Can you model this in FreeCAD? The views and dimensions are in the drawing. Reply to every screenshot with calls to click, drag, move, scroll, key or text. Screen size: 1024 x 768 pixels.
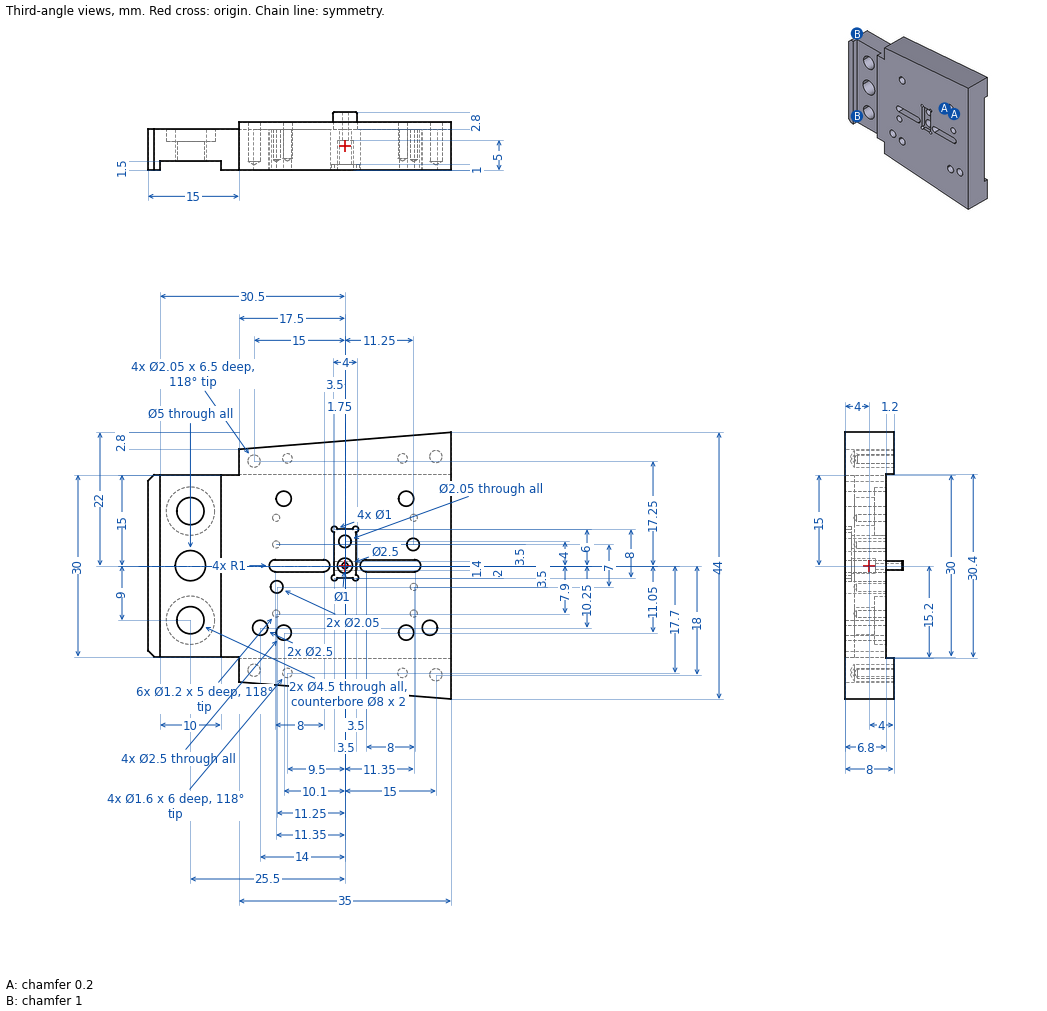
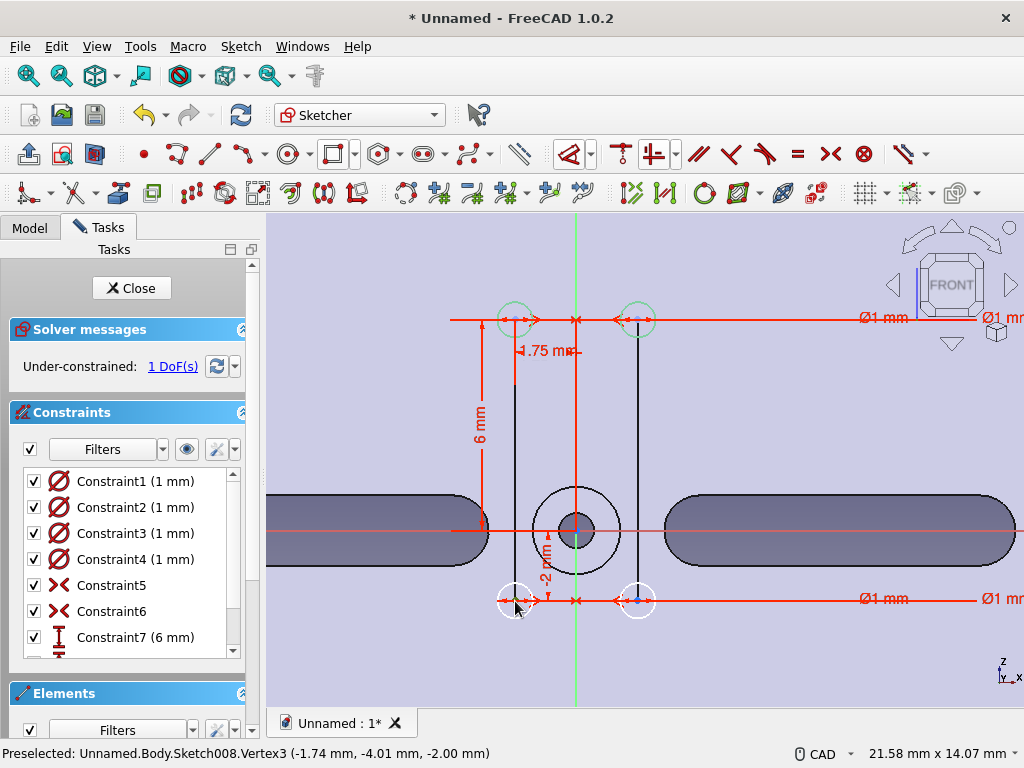
key(l)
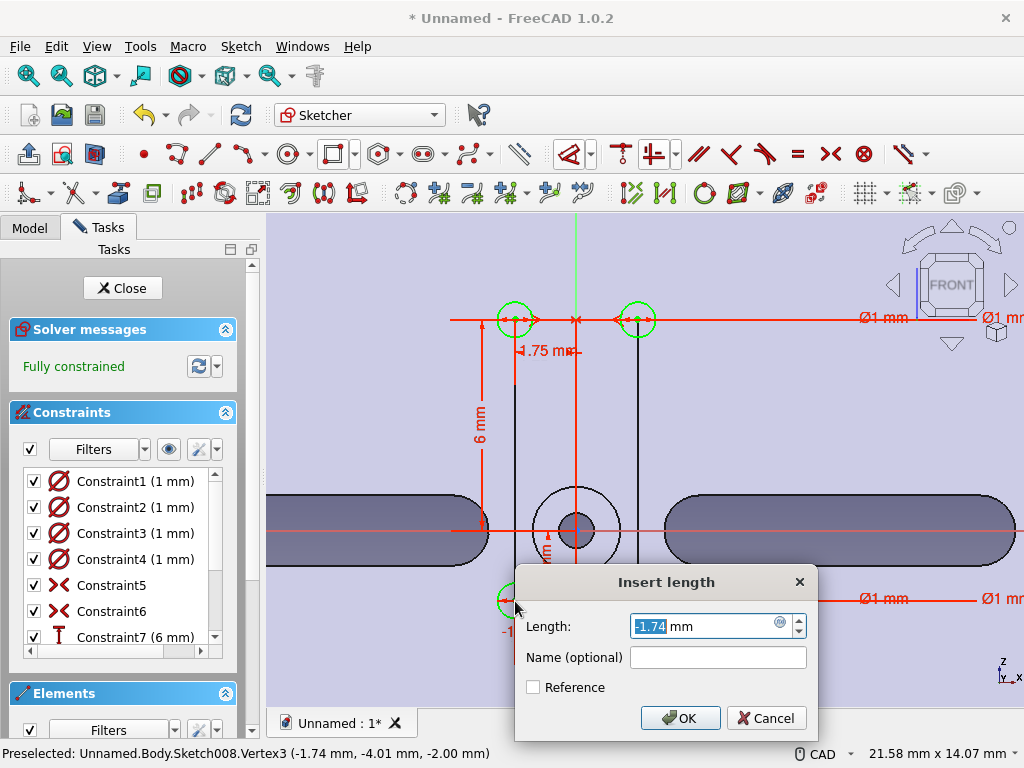
text(-1.75)
key(Return)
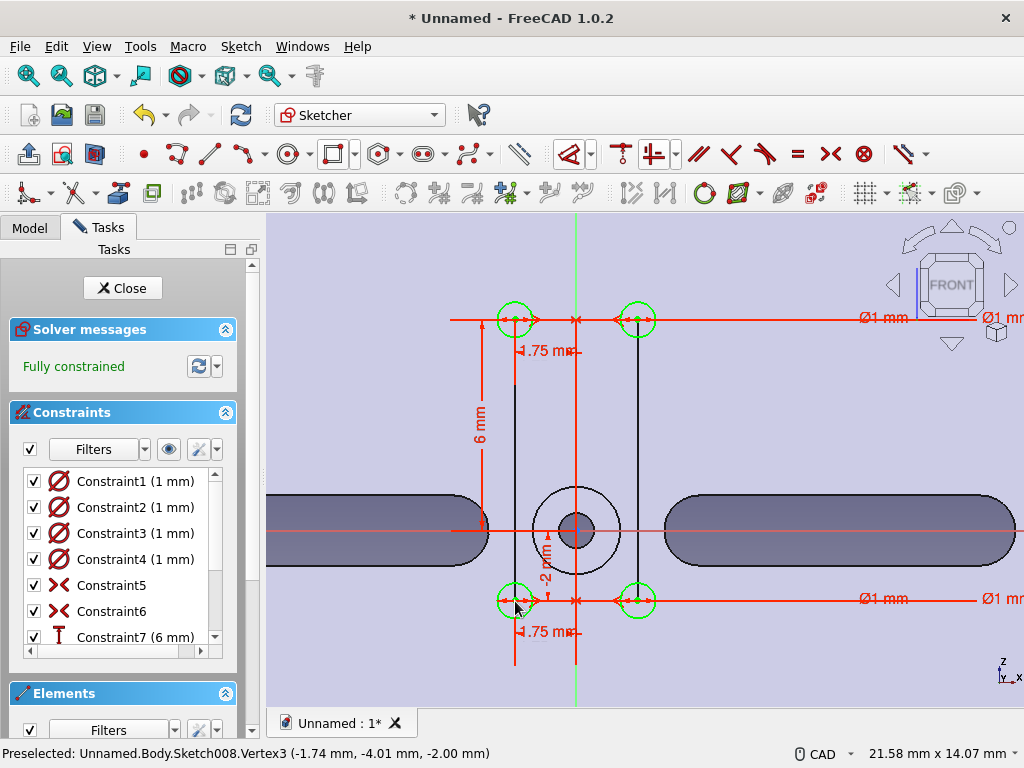
click(123, 288)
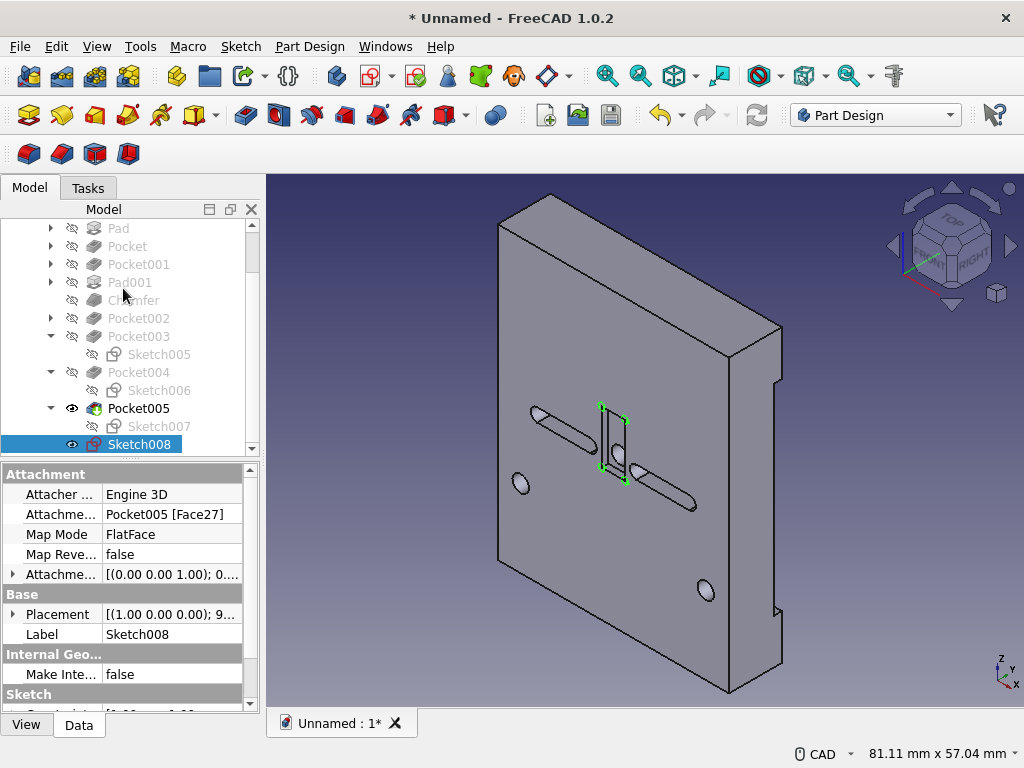
click(246, 116)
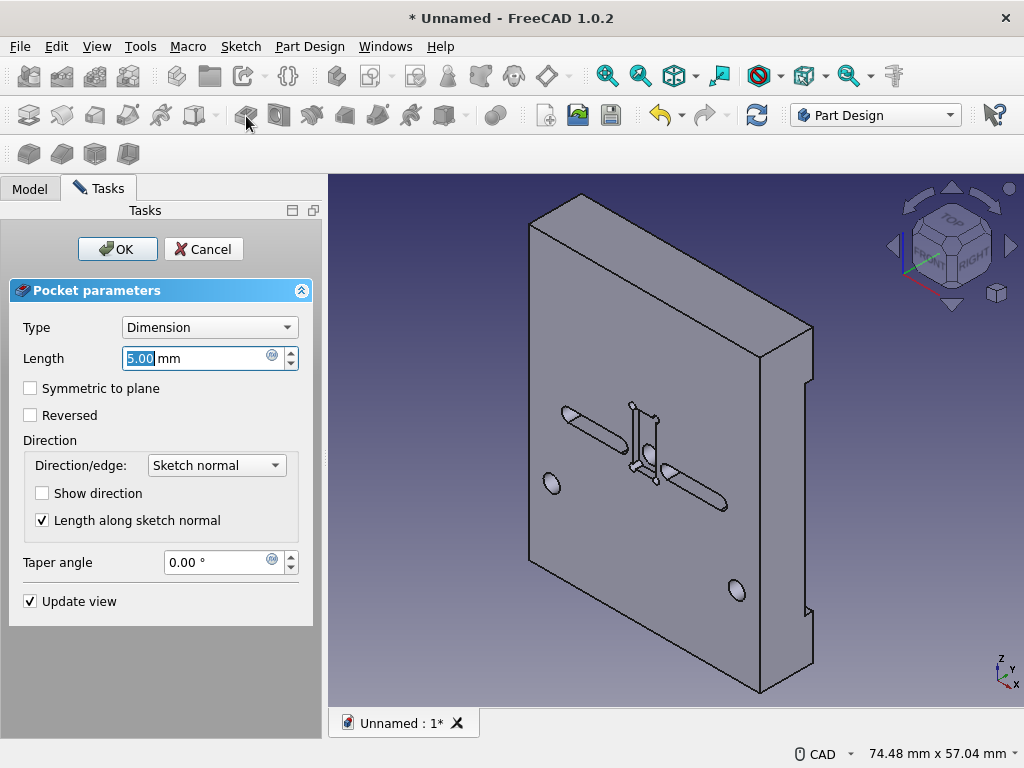
text(1)
key(Tab)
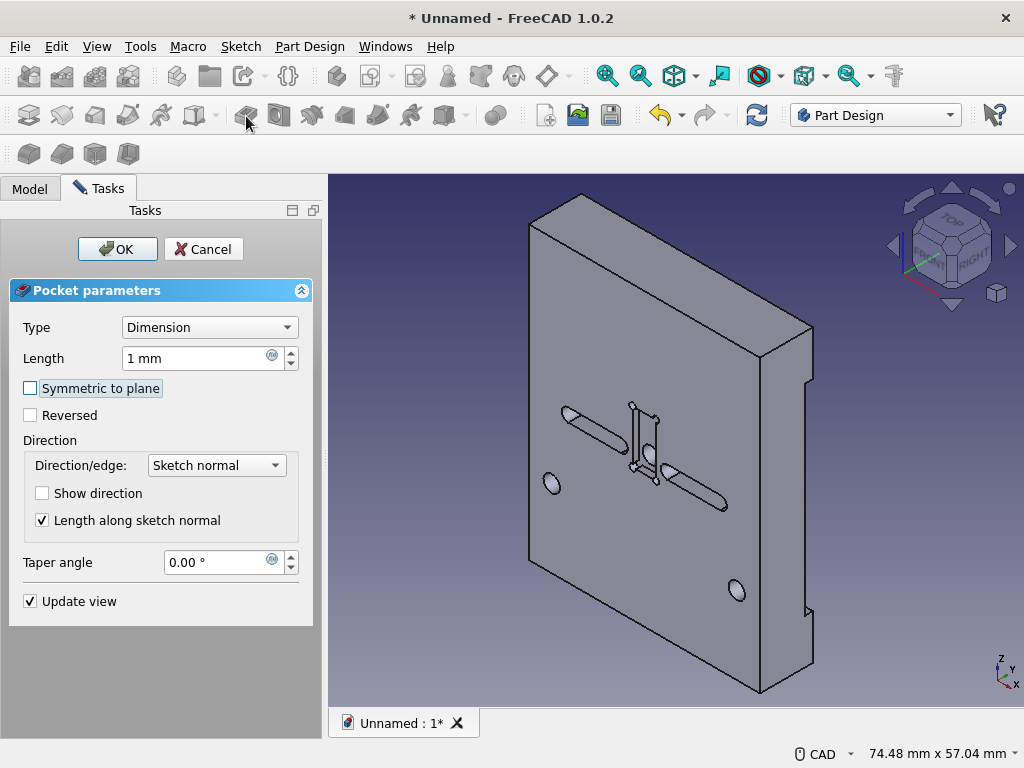
click(118, 249)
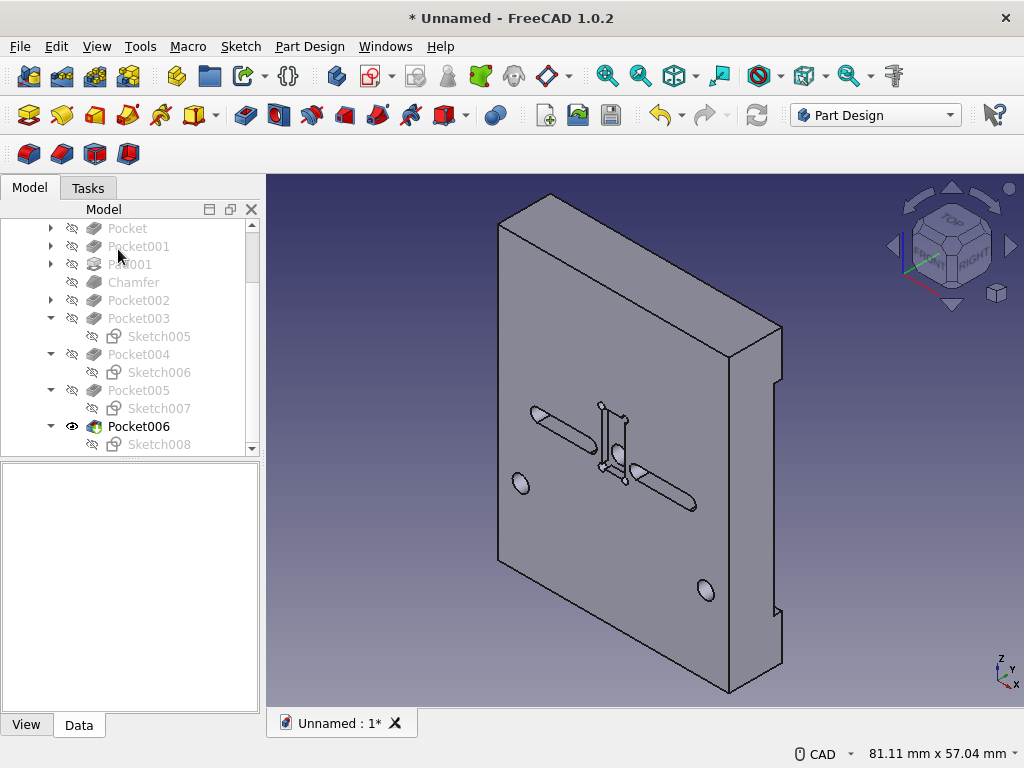
click(616, 426)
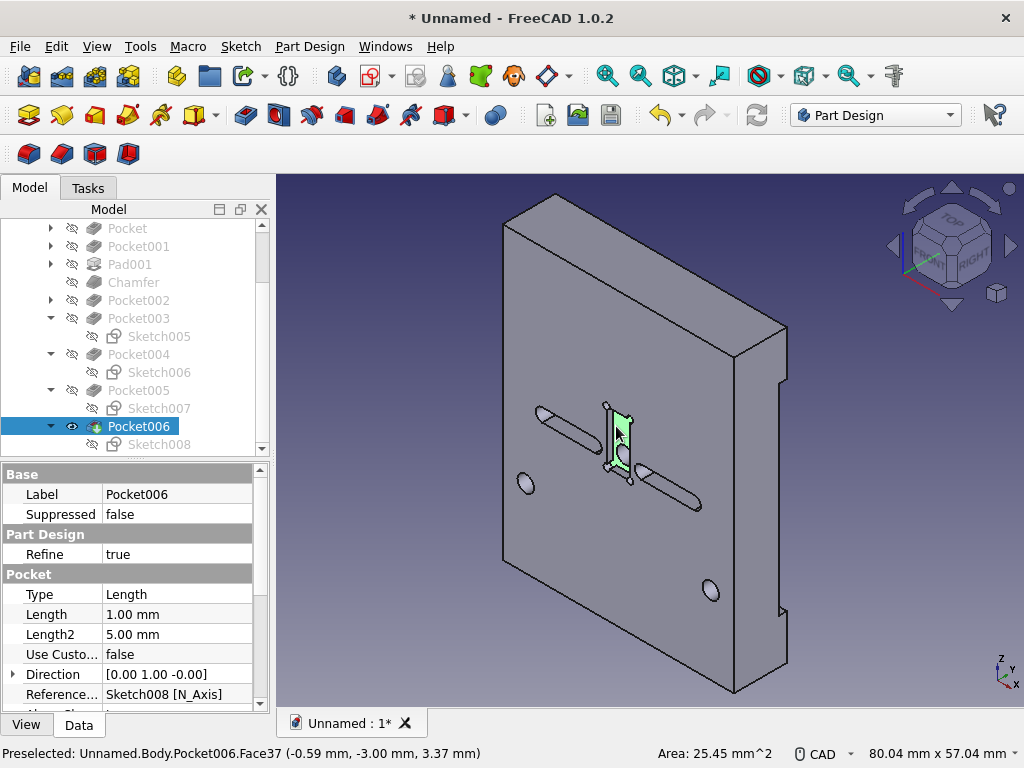
click(370, 76)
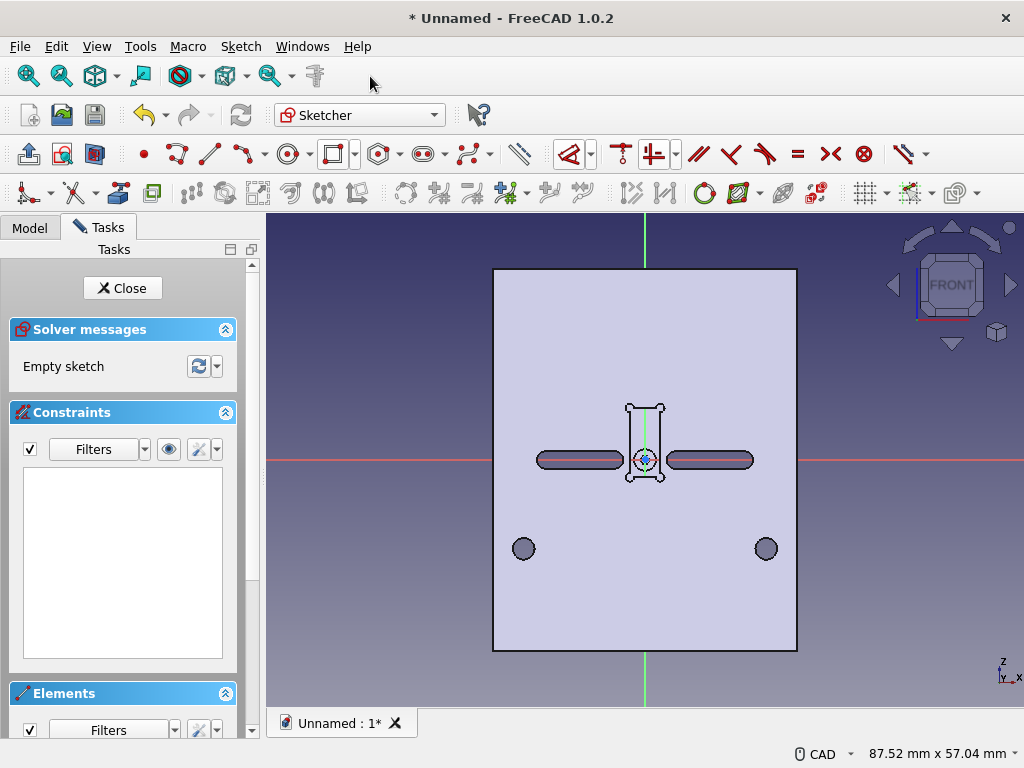
scroll(656, 435, up, 10)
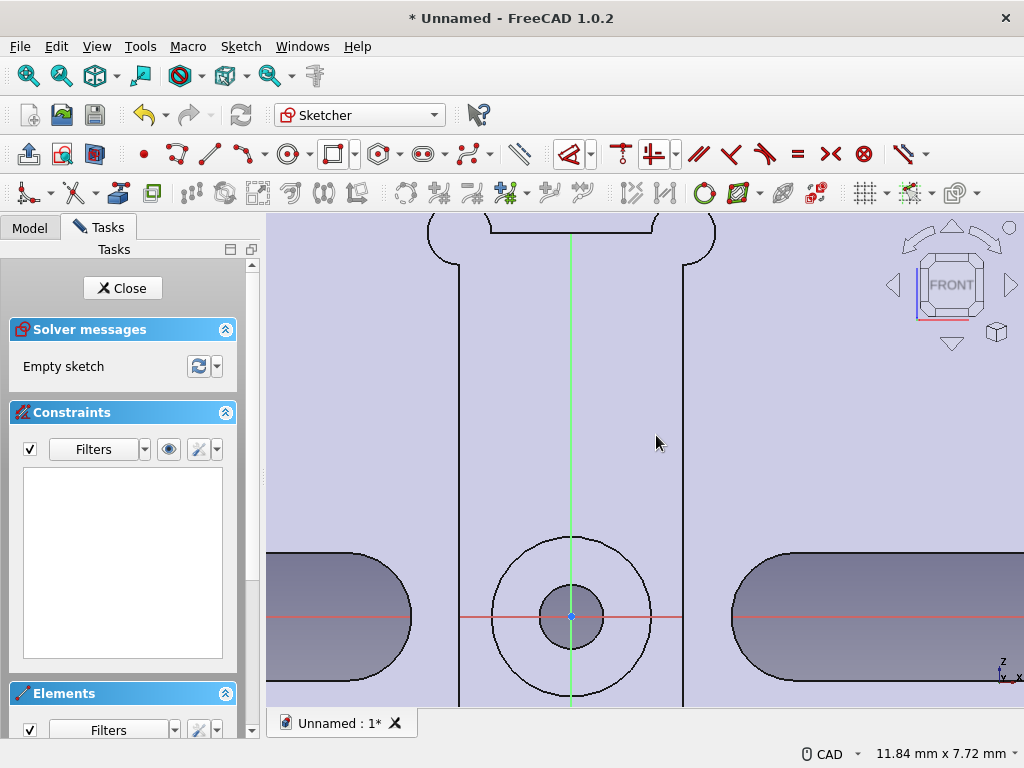
click(288, 154)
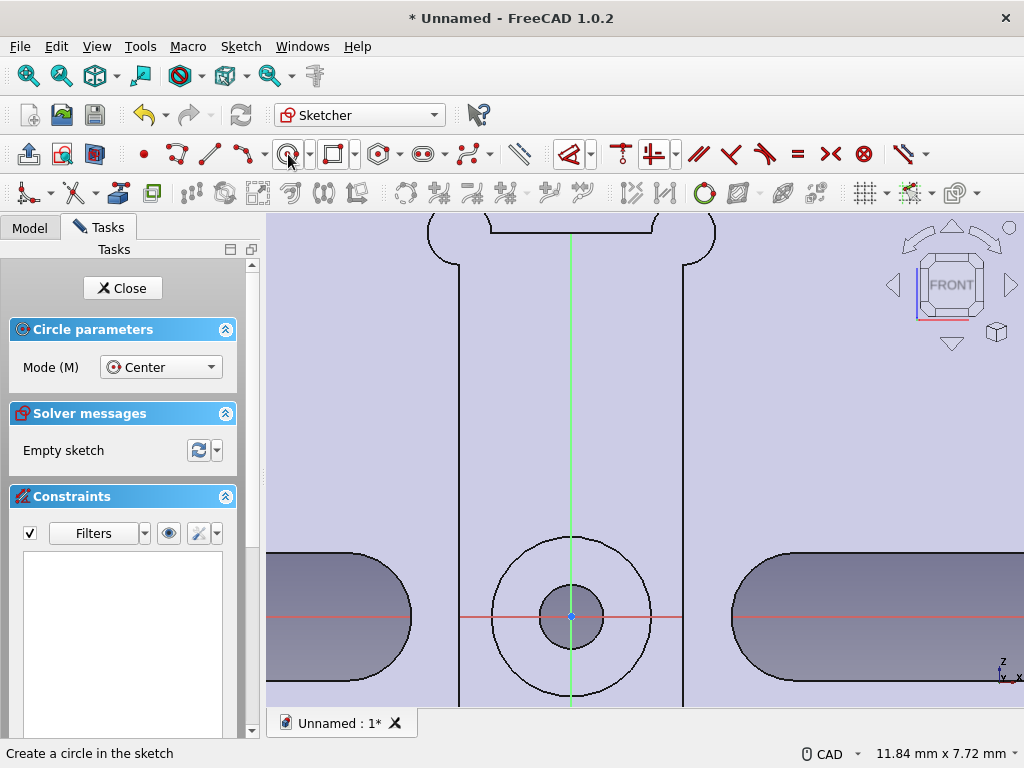
click(571, 361)
move(618, 314)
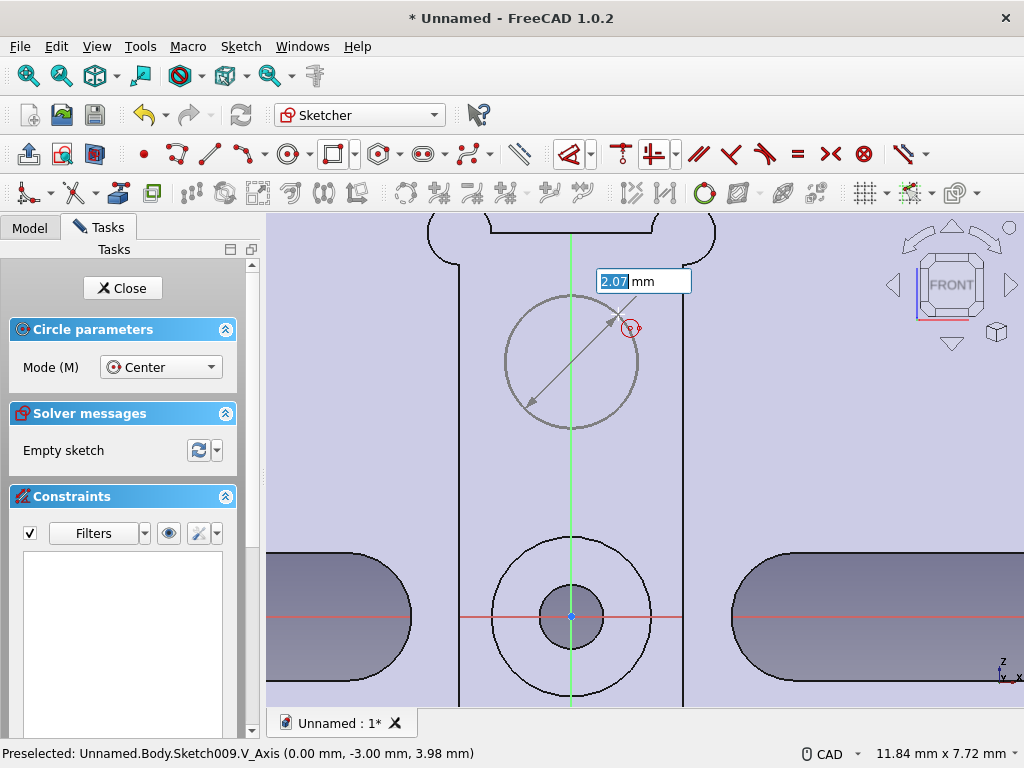
text(2.05)
key(Return)
key(Escape)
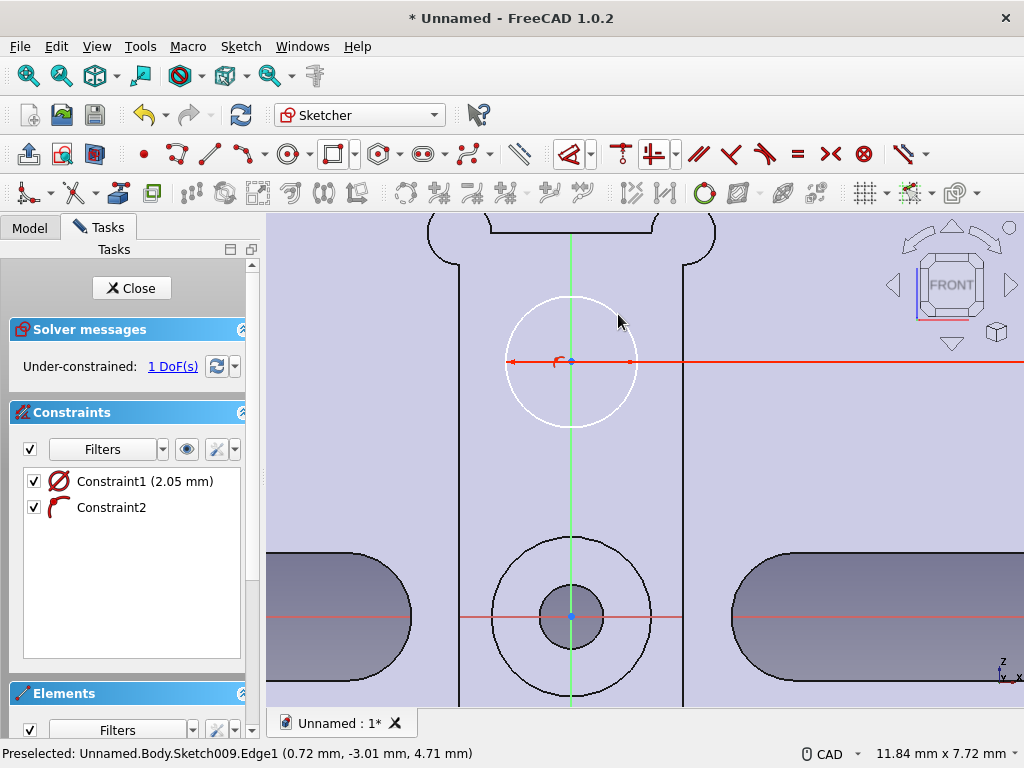
click(571, 362)